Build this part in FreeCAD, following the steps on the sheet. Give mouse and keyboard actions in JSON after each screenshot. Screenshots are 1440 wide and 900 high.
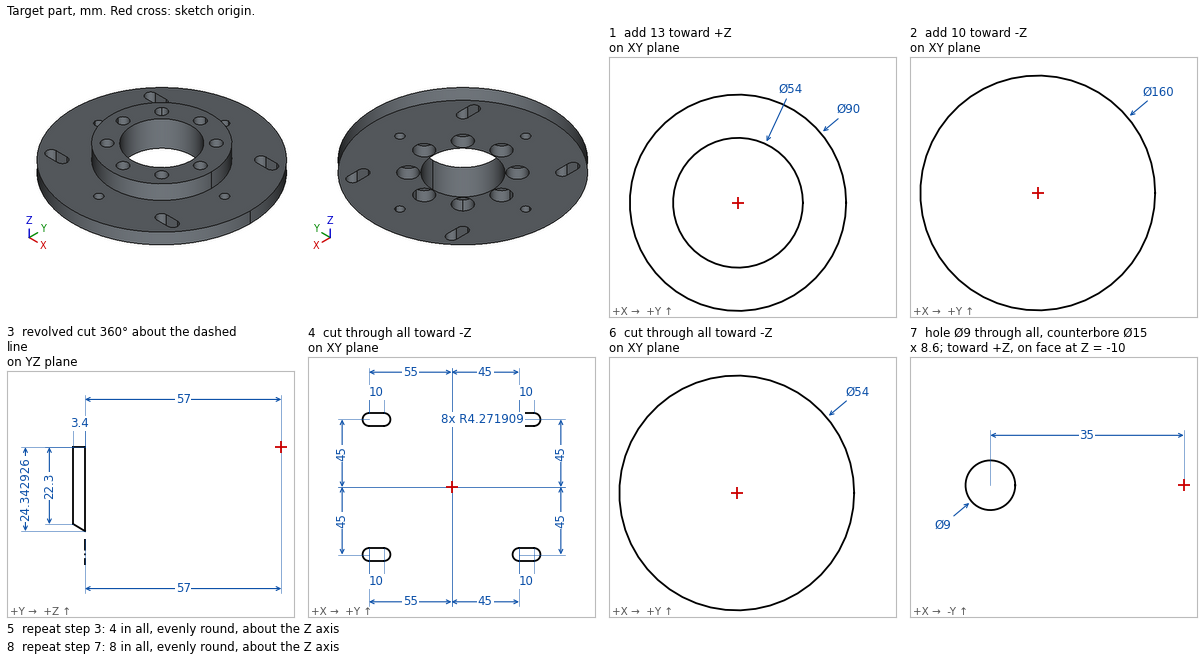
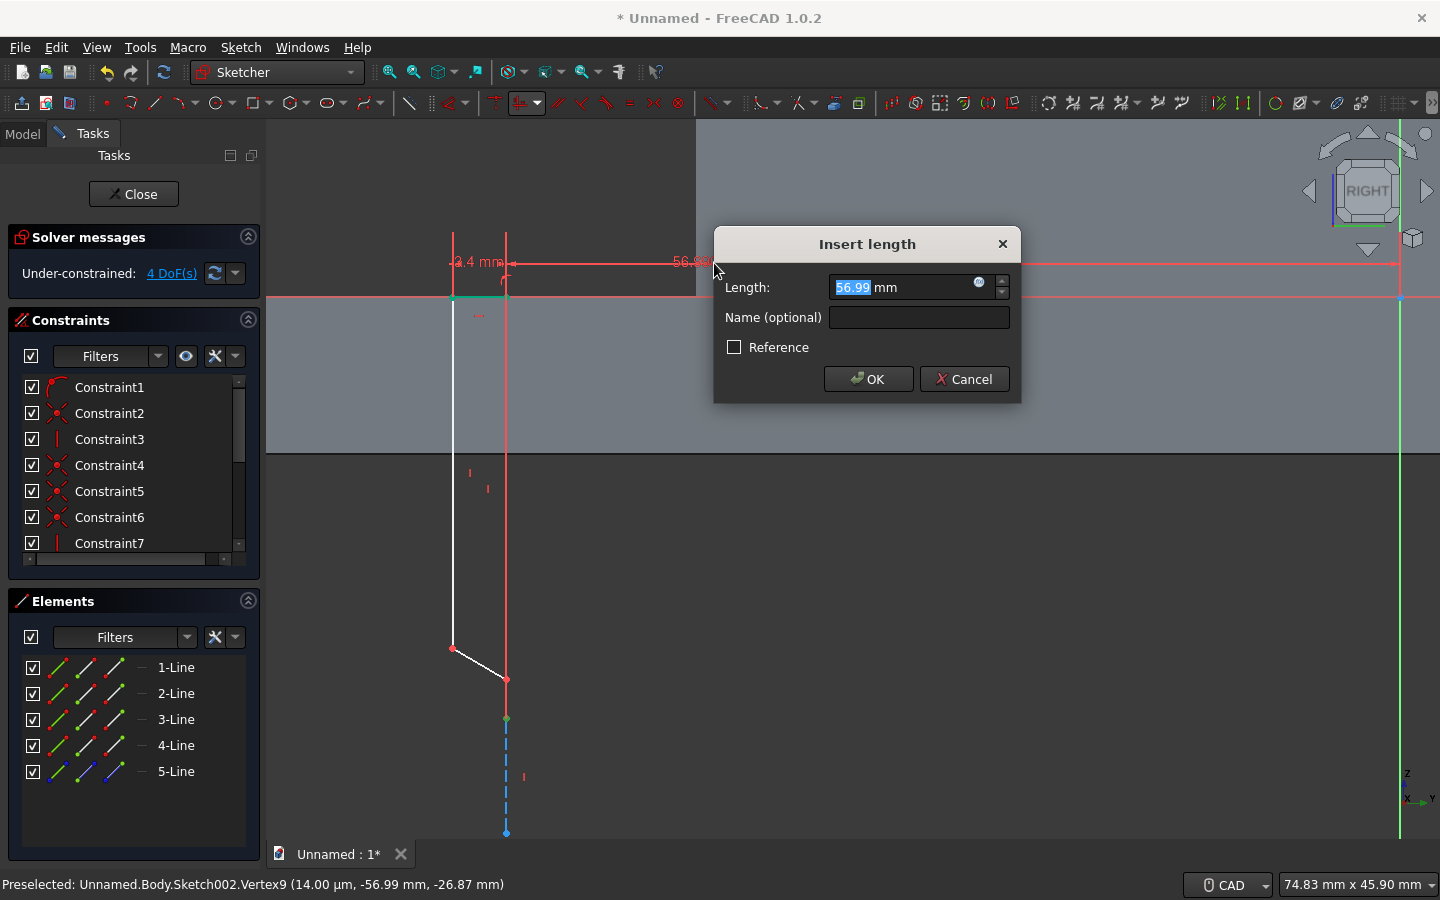
{"action": "type", "text": "57"}
{"action": "key", "text": "Return"}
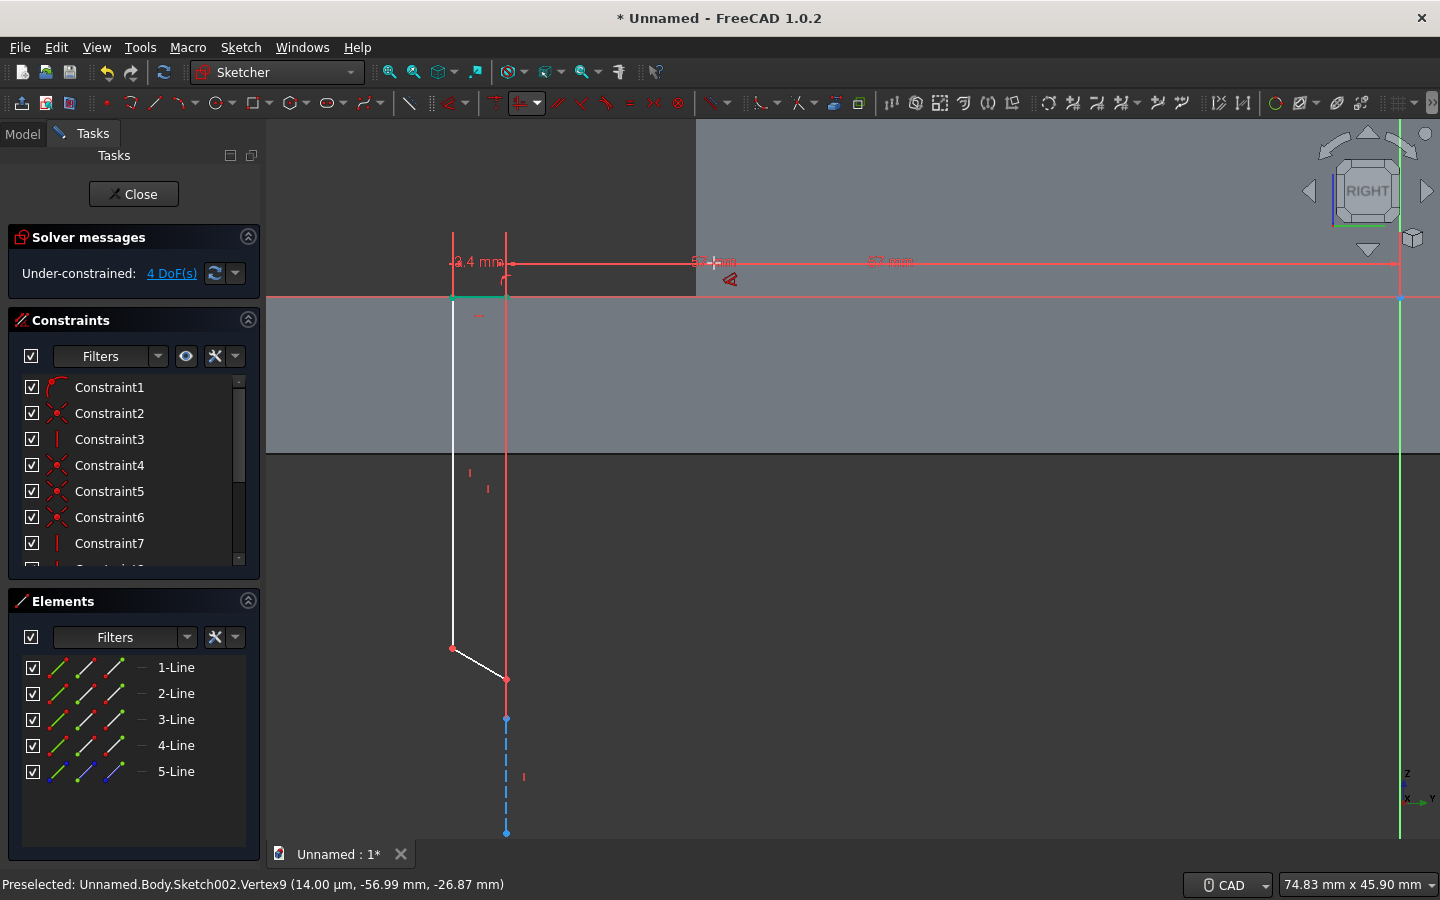
{"action": "left_click", "coordinate": [453, 402]}
{"action": "left_click", "coordinate": [419, 473]}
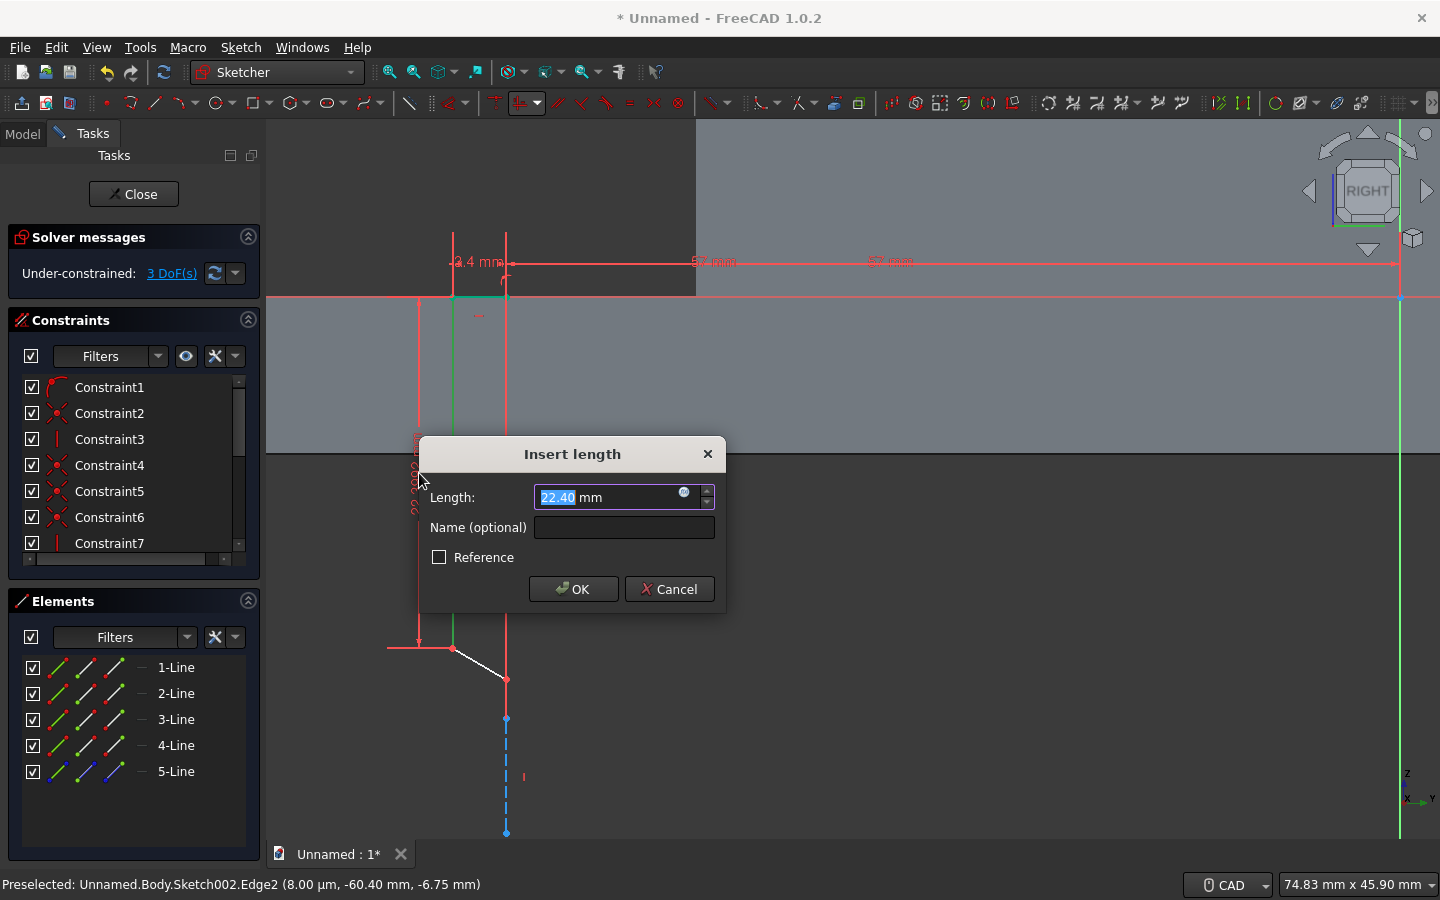
{"action": "type", "text": "22.3"}
{"action": "key", "text": "Return"}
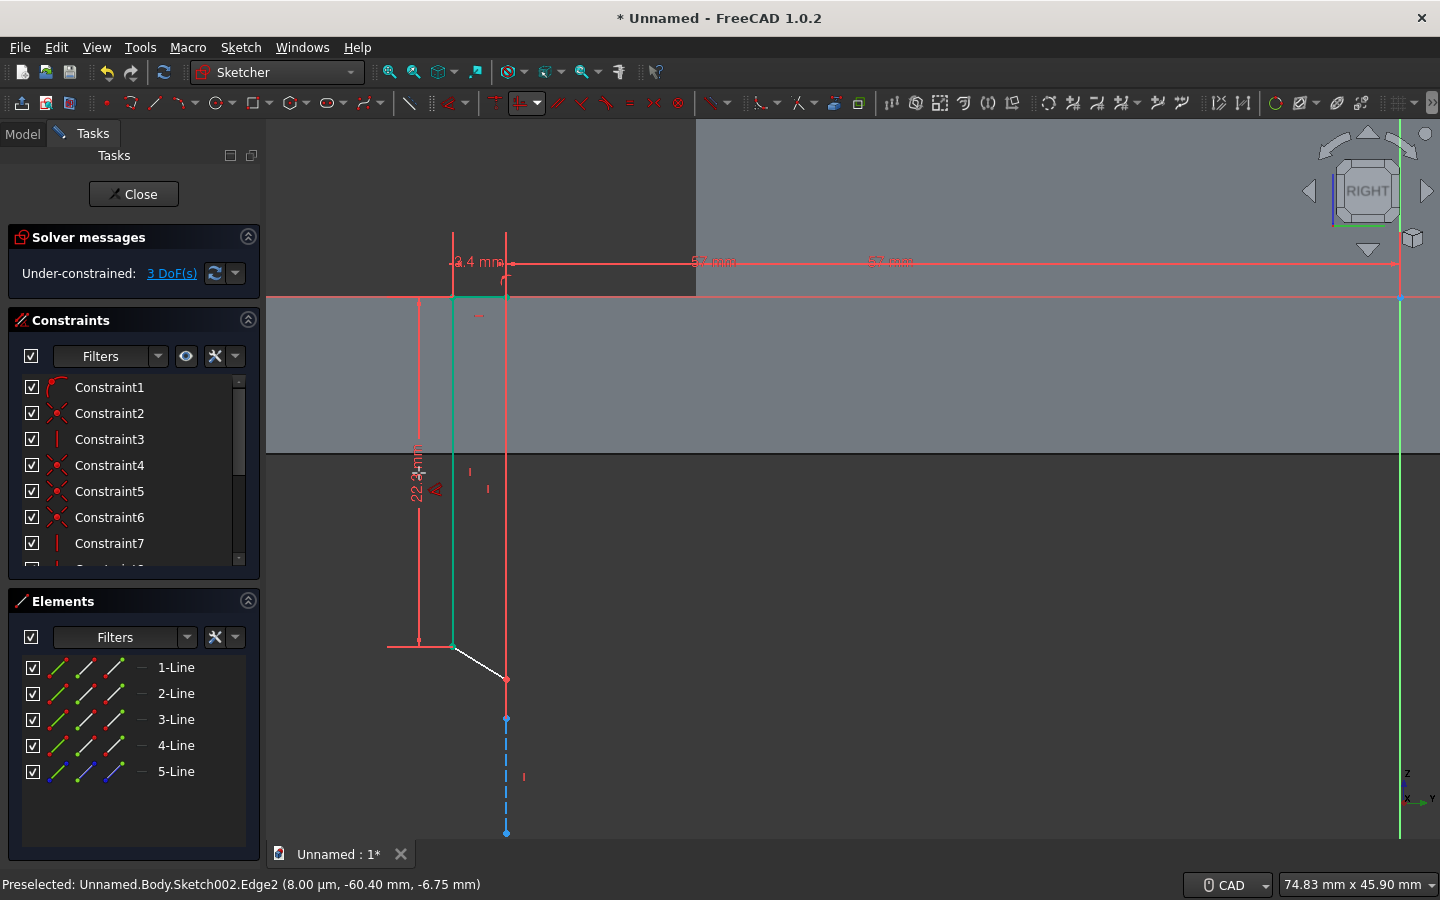
{"action": "left_click", "coordinate": [506, 565]}
{"action": "left_click", "coordinate": [472, 400]}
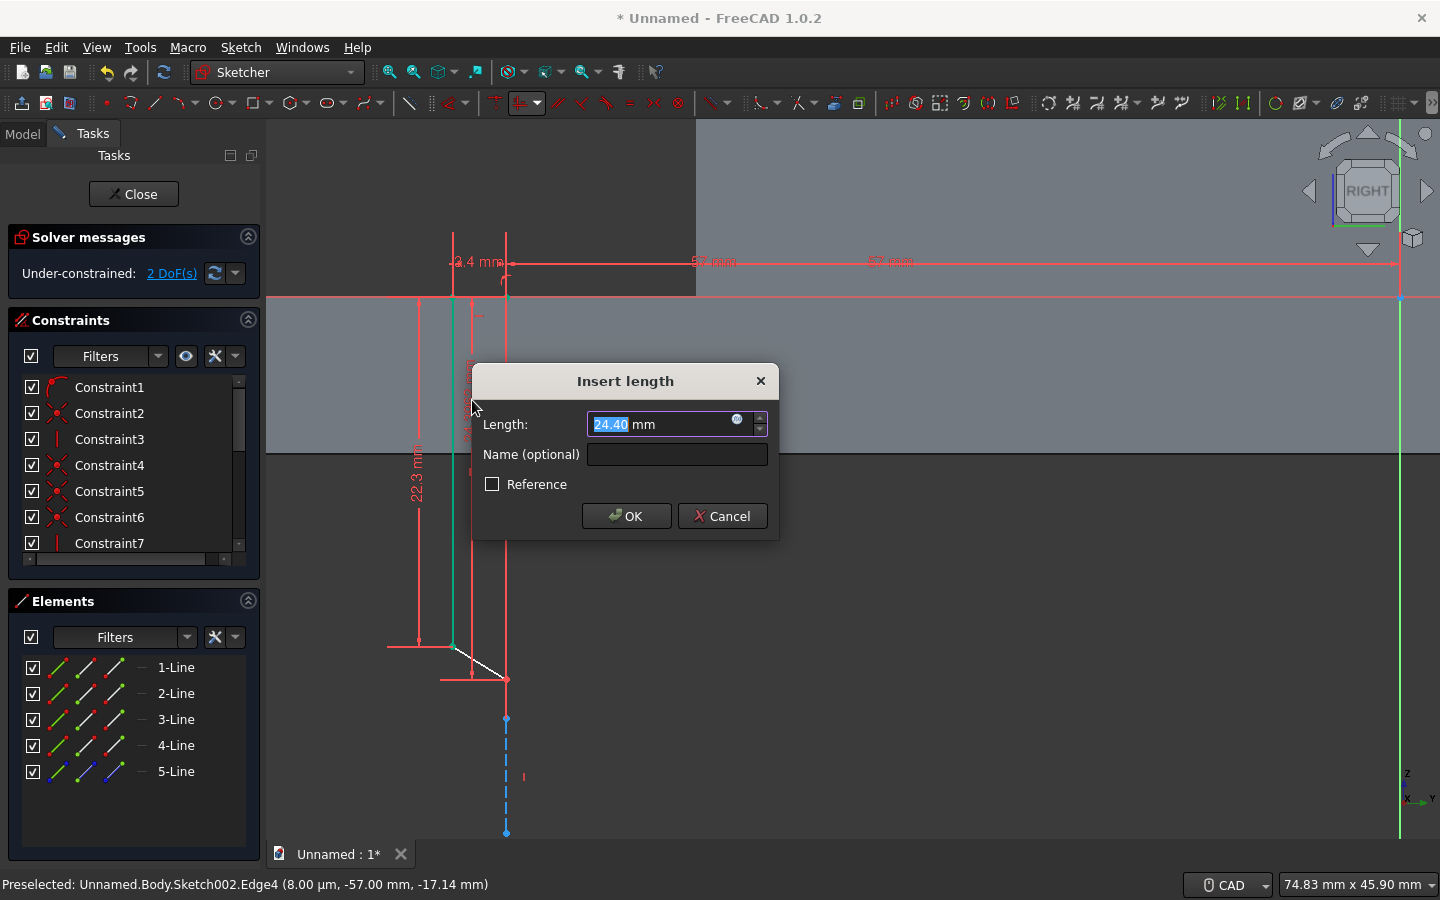
{"action": "type", "text": "24.342926"}
{"action": "key", "text": "Return"}
{"action": "key", "text": "Escape"}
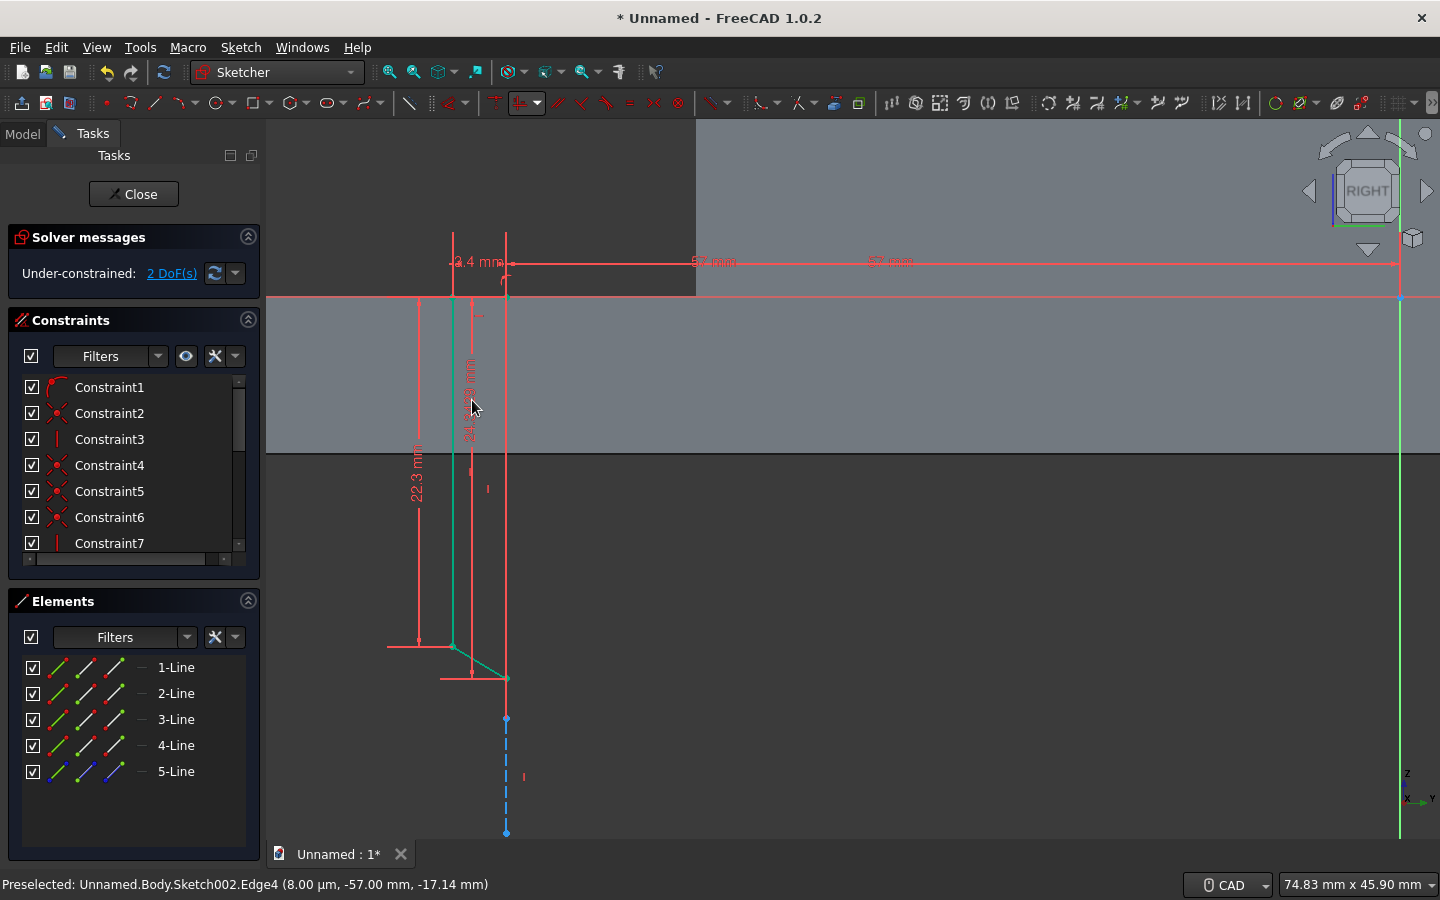
{"action": "left_click", "coordinate": [134, 194]}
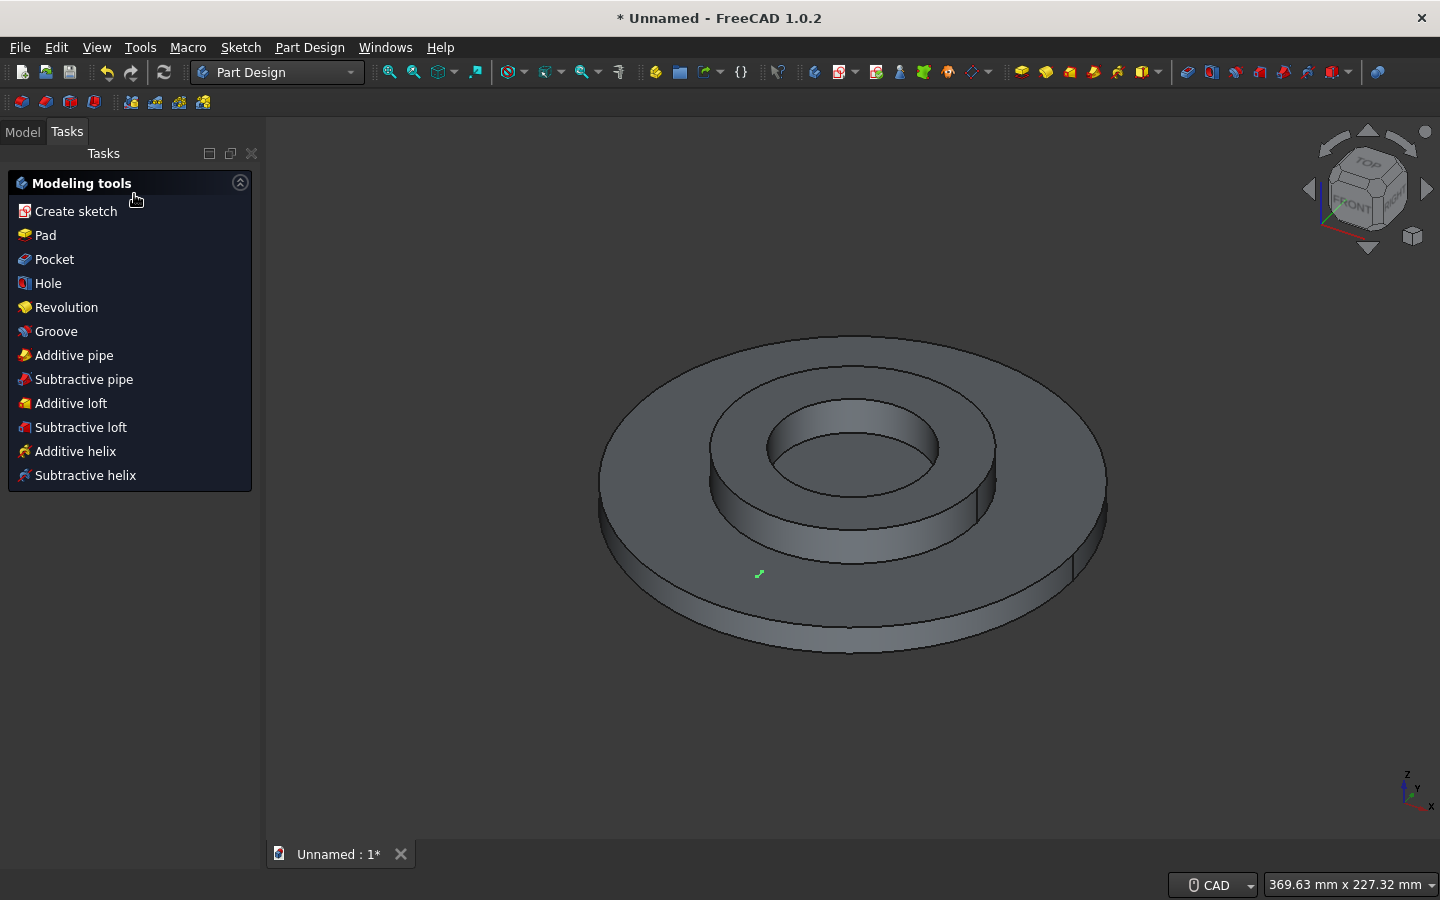
{"action": "left_click", "coordinate": [1236, 72]}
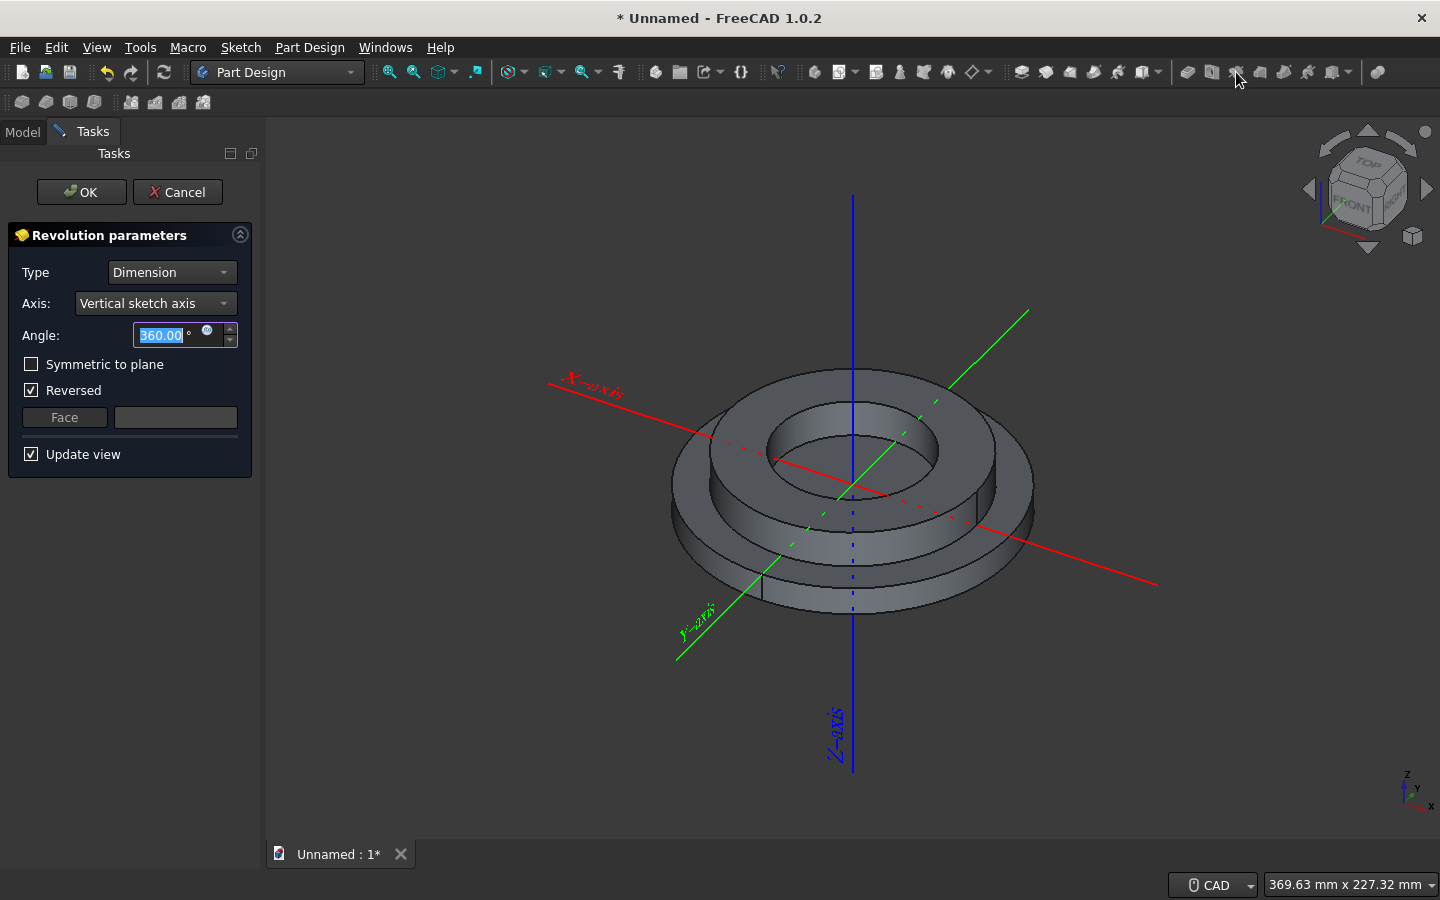
{"action": "left_click", "coordinate": [156, 304]}